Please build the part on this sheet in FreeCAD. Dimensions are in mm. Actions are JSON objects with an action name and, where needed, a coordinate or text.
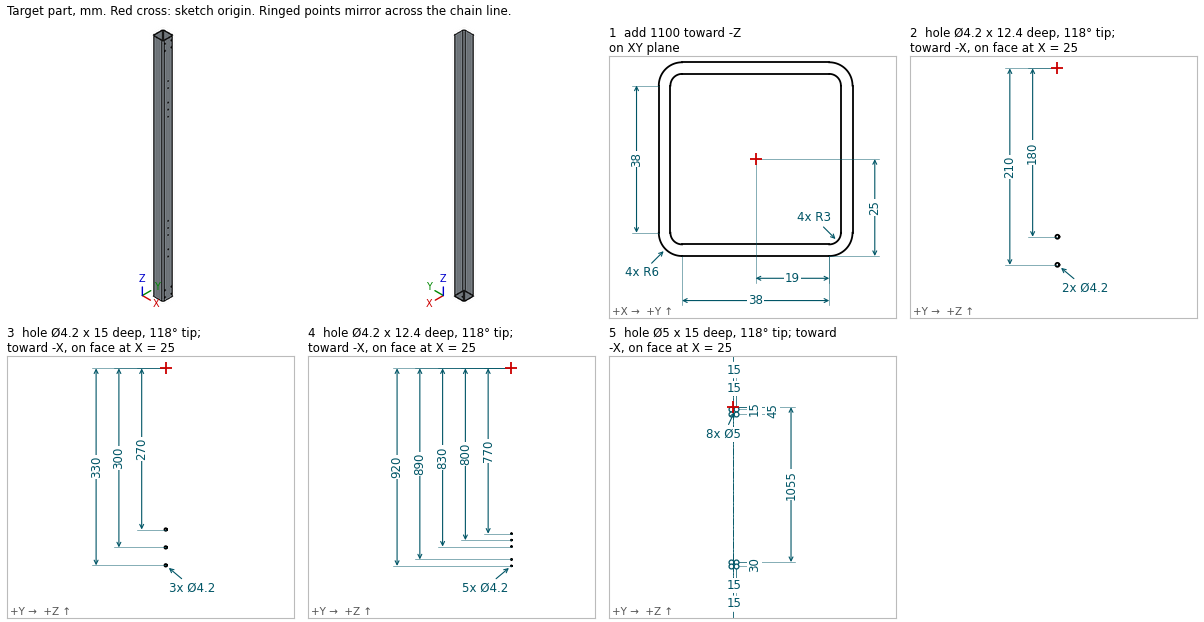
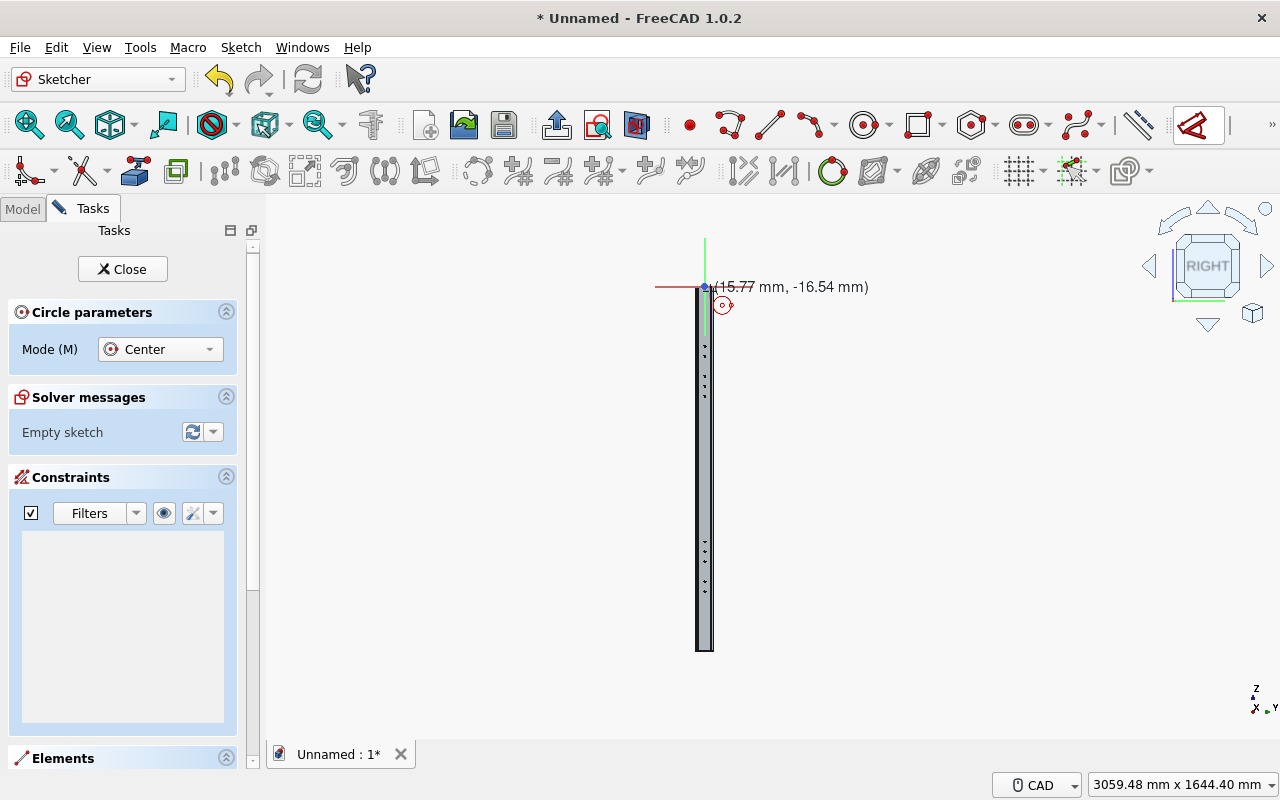
{"action": "scroll", "coordinate": [710, 291], "scroll_direction": "up", "scroll_amount": 6}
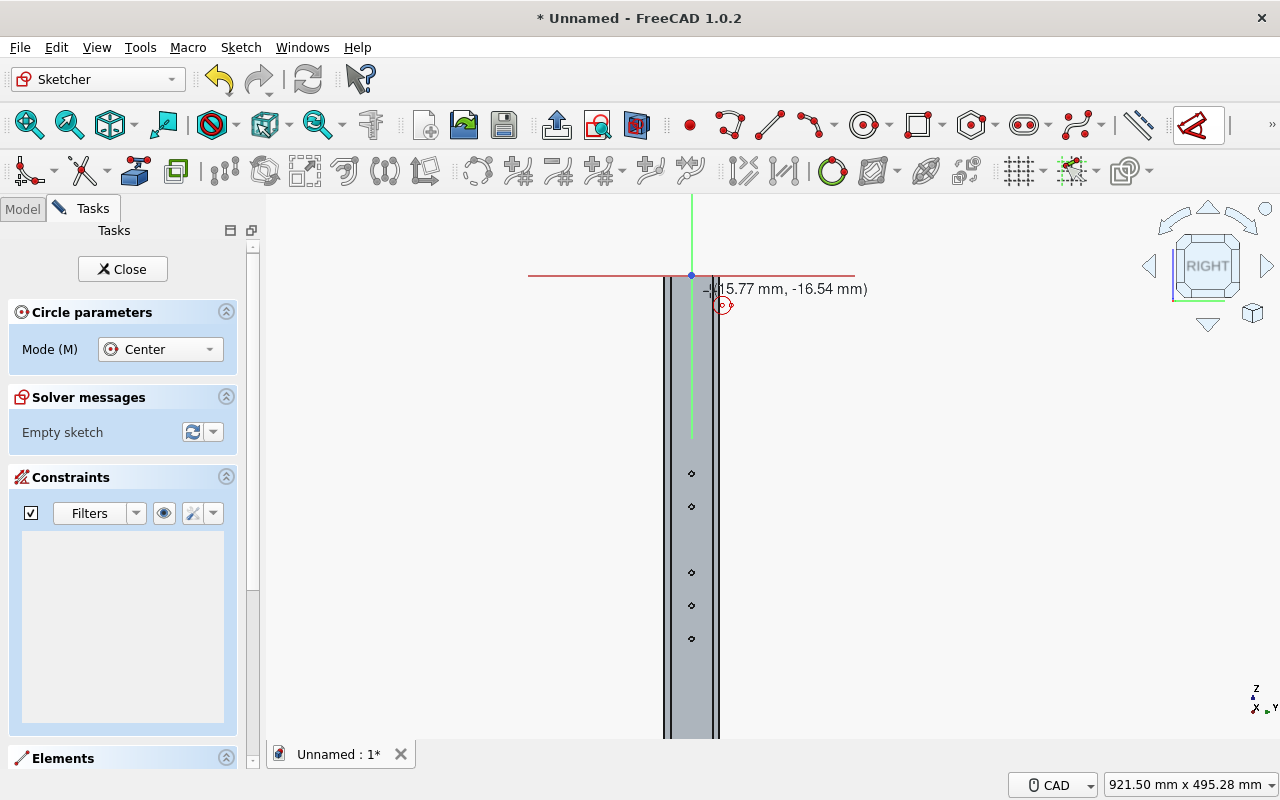
{"action": "left_click", "coordinate": [708, 292]}
{"action": "mouse_move", "coordinate": [710, 290]}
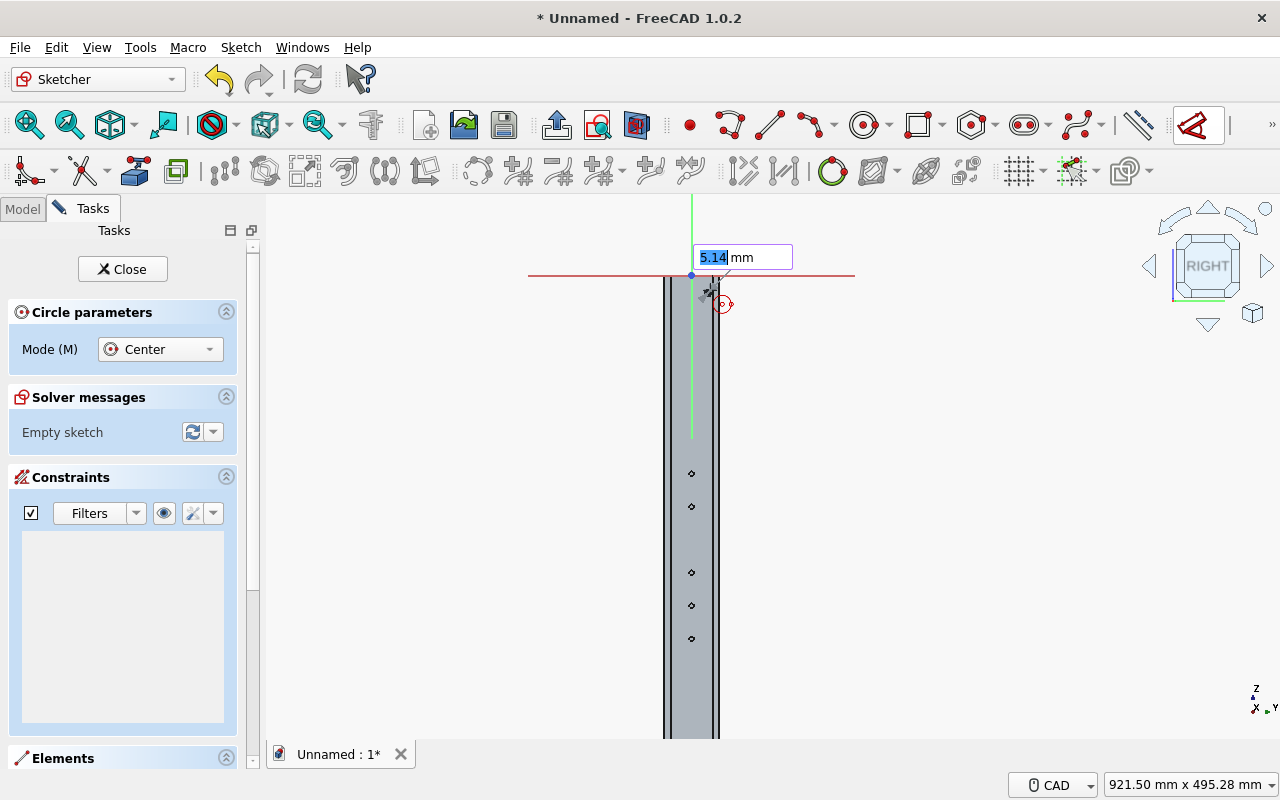
{"action": "type", "text": "5"}
{"action": "key", "text": "Return"}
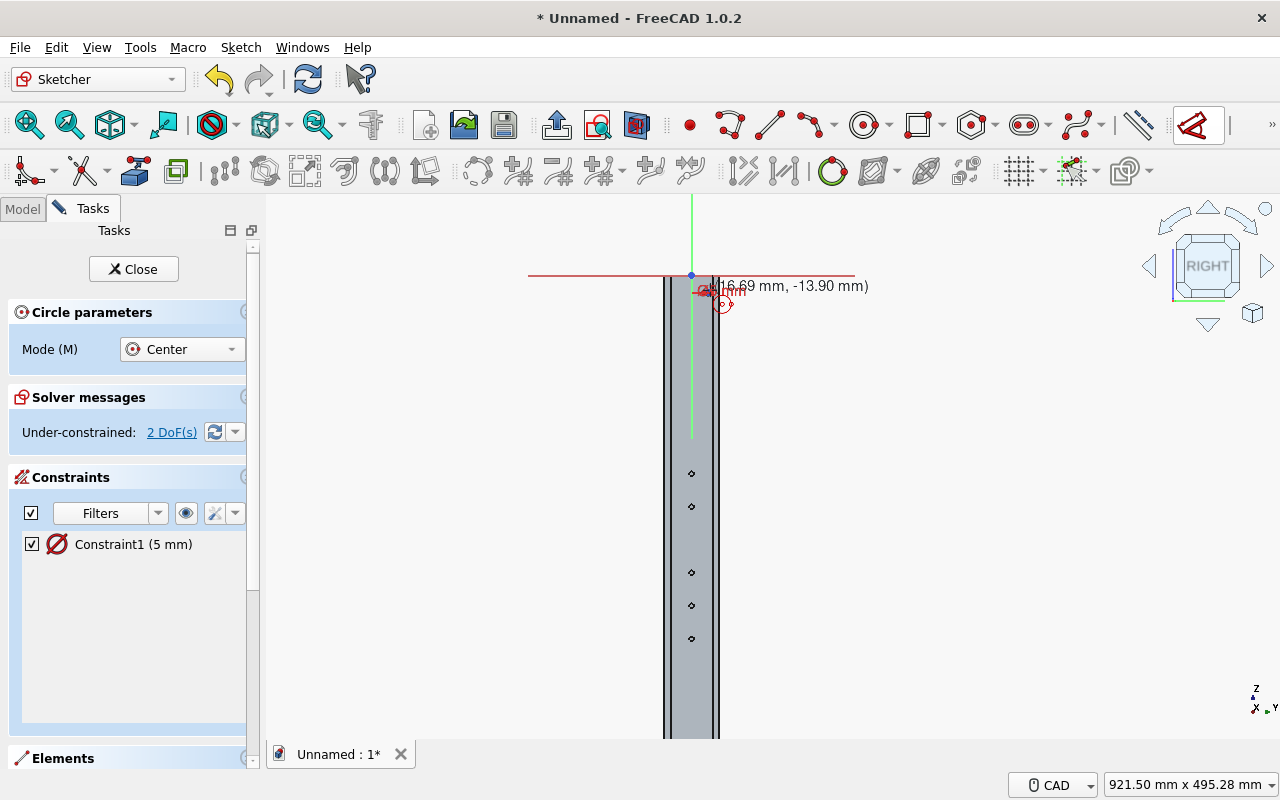
{"action": "scroll", "coordinate": [708, 325], "scroll_direction": "up", "scroll_amount": 11}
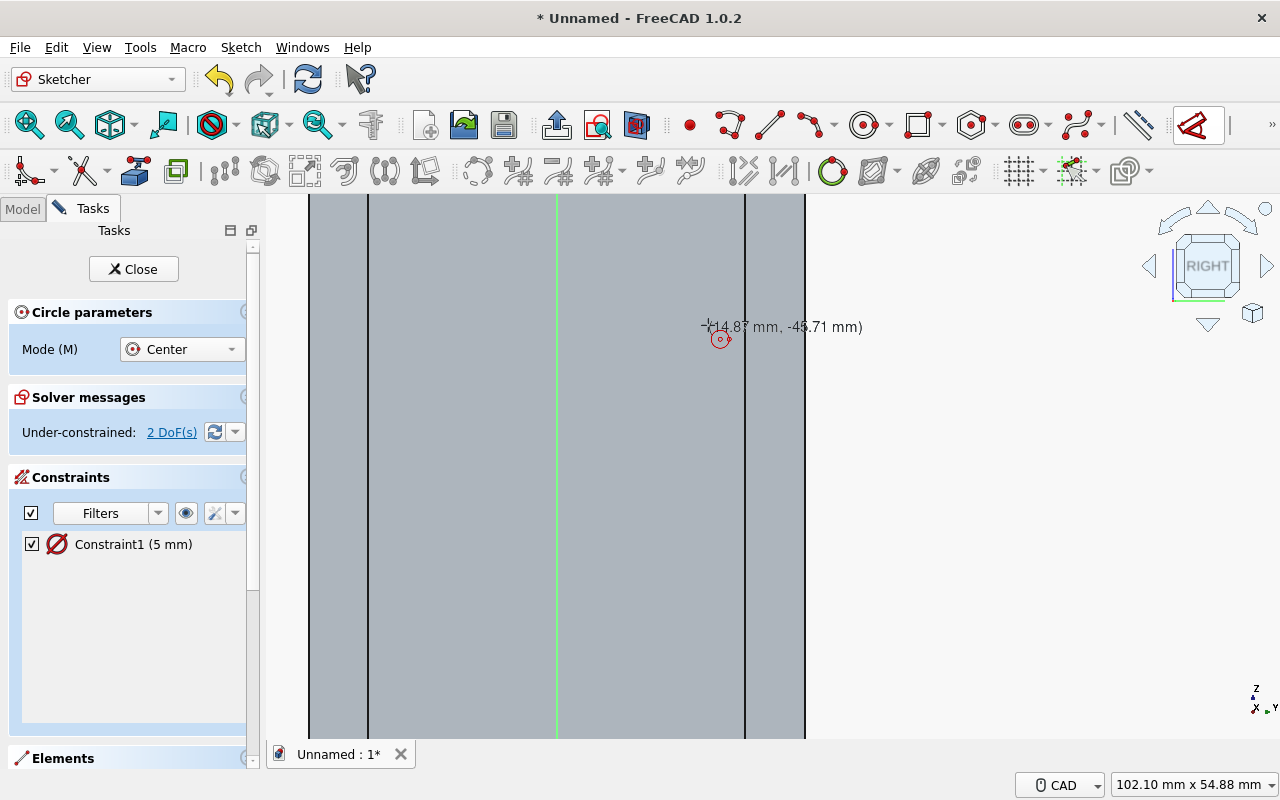
{"action": "scroll", "coordinate": [710, 300], "scroll_direction": "down", "scroll_amount": 17}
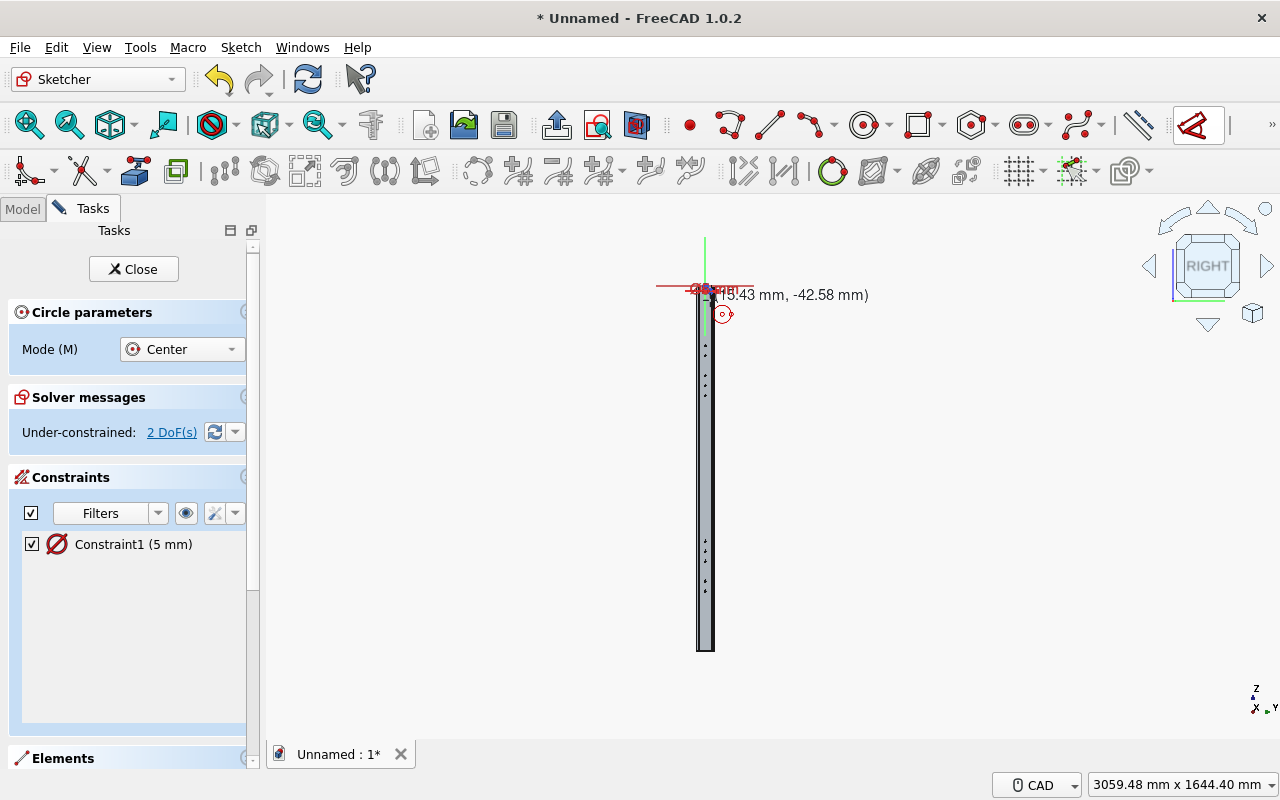
{"action": "scroll", "coordinate": [710, 301], "scroll_direction": "up", "scroll_amount": 6}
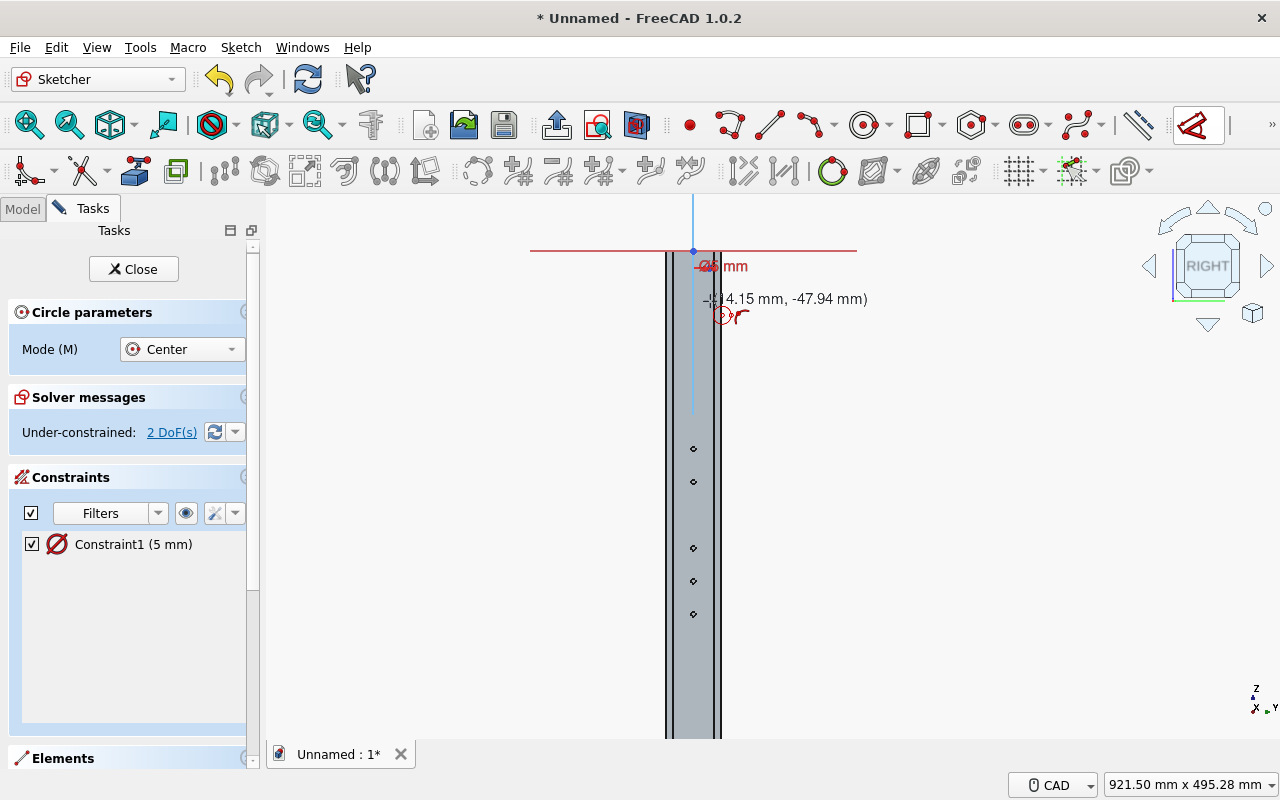
{"action": "left_click", "coordinate": [710, 301]}
{"action": "mouse_move", "coordinate": [712, 299]}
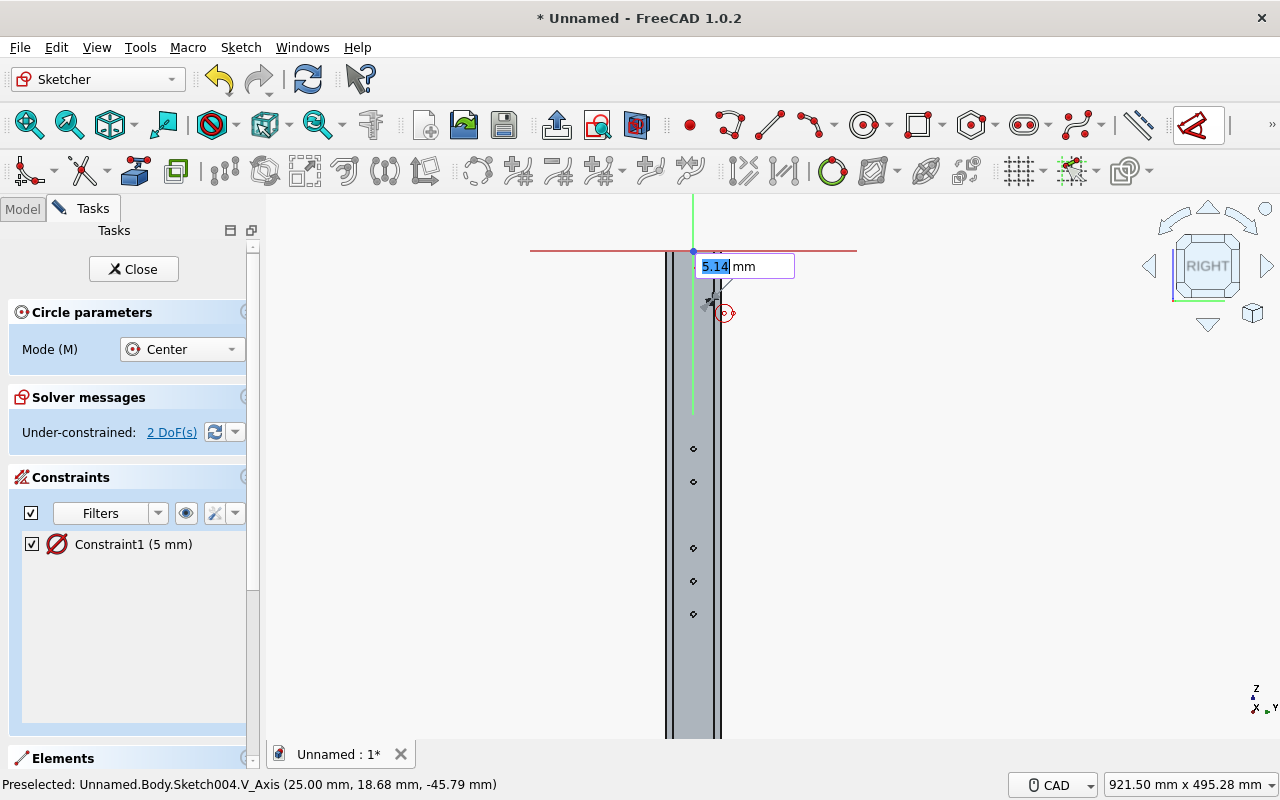
{"action": "type", "text": "5"}
{"action": "key", "text": "Return"}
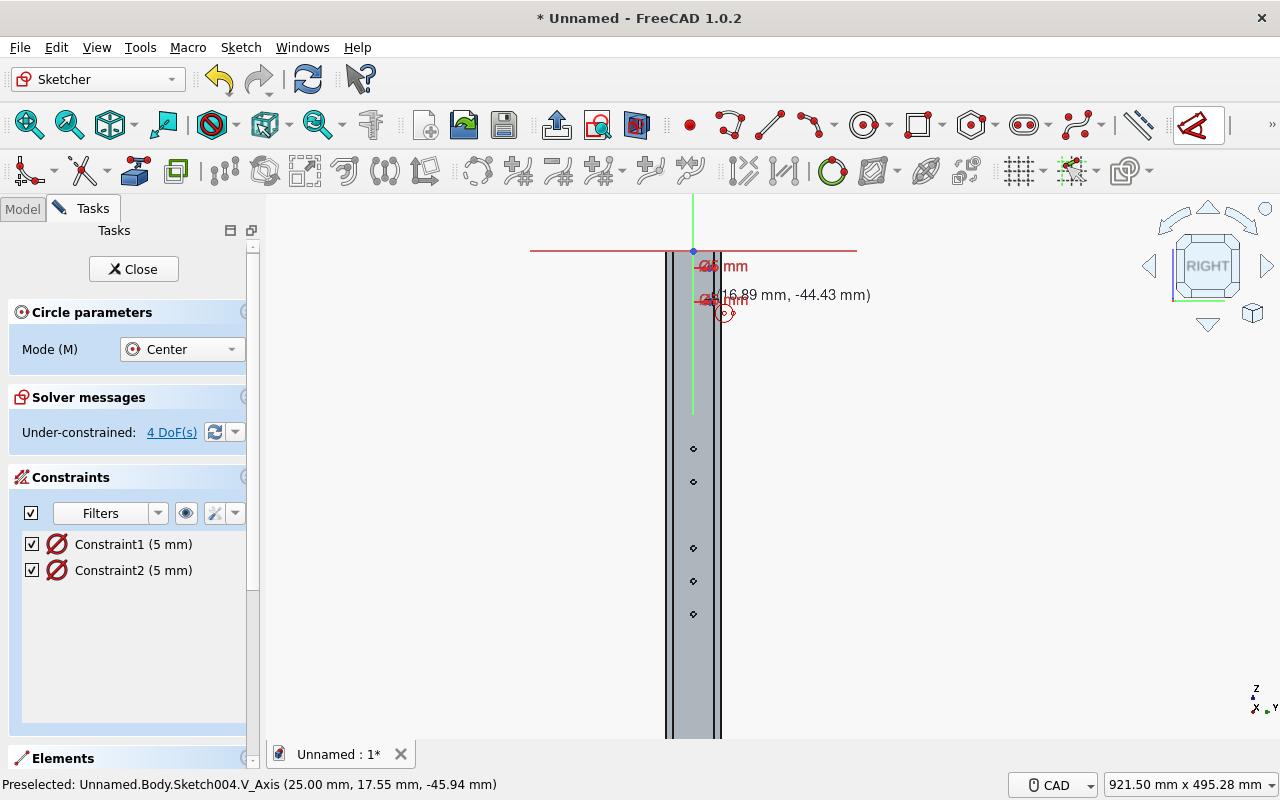
{"action": "scroll", "coordinate": [677, 268], "scroll_direction": "up", "scroll_amount": 11}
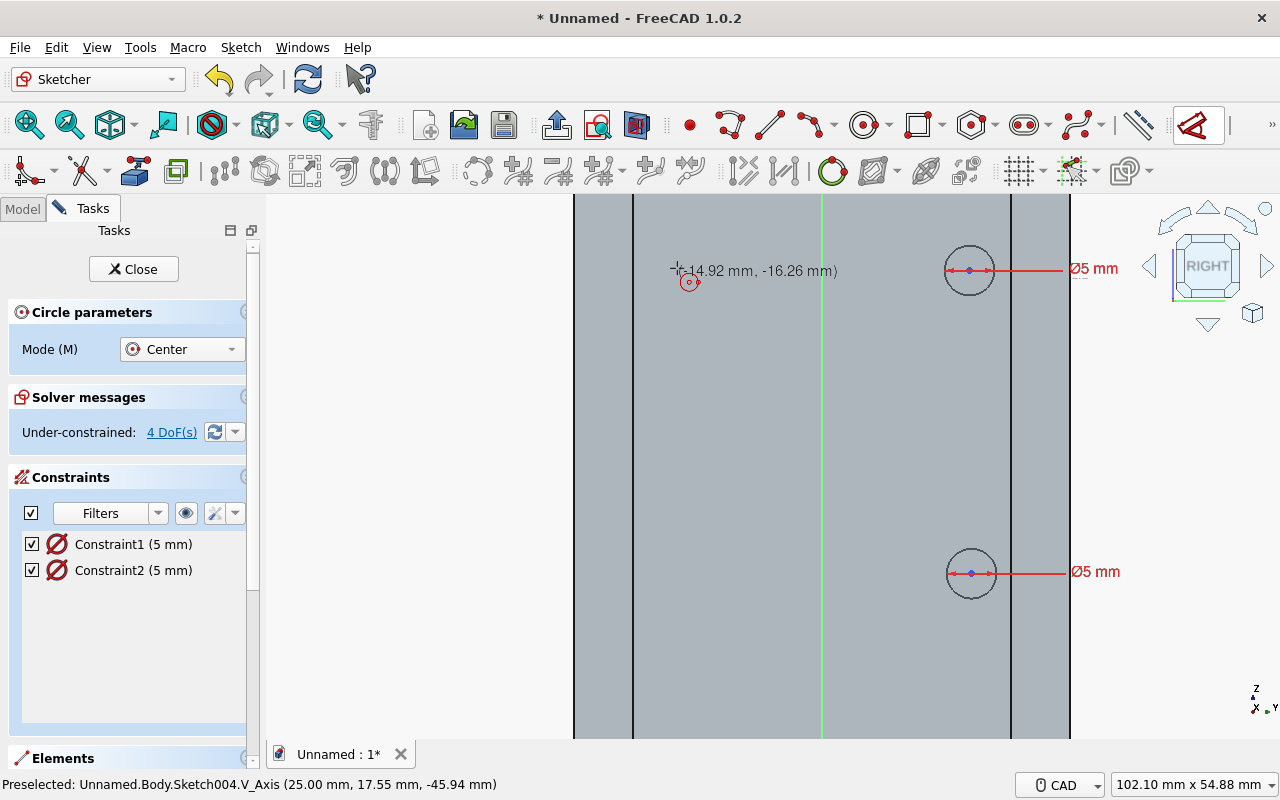
{"action": "scroll", "coordinate": [700, 292], "scroll_direction": "down", "scroll_amount": 17}